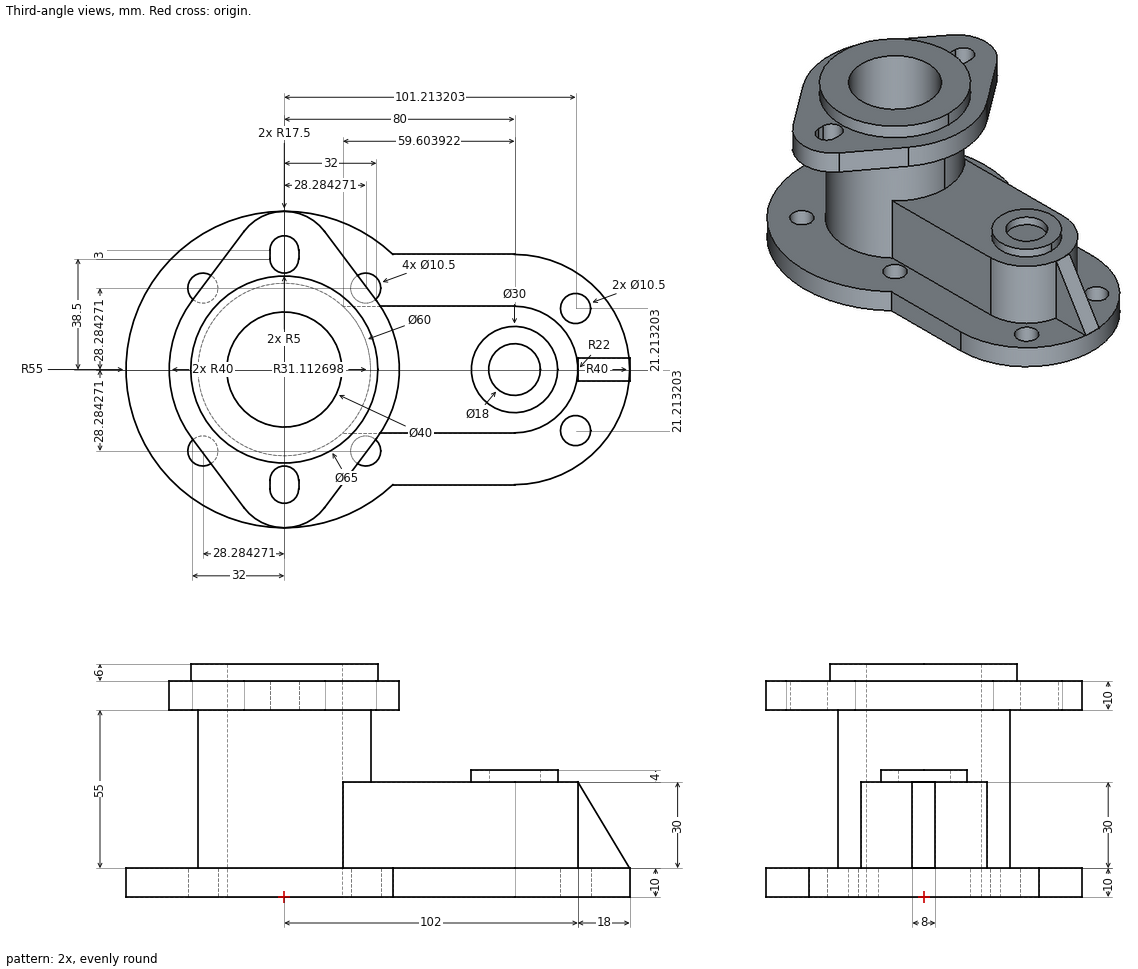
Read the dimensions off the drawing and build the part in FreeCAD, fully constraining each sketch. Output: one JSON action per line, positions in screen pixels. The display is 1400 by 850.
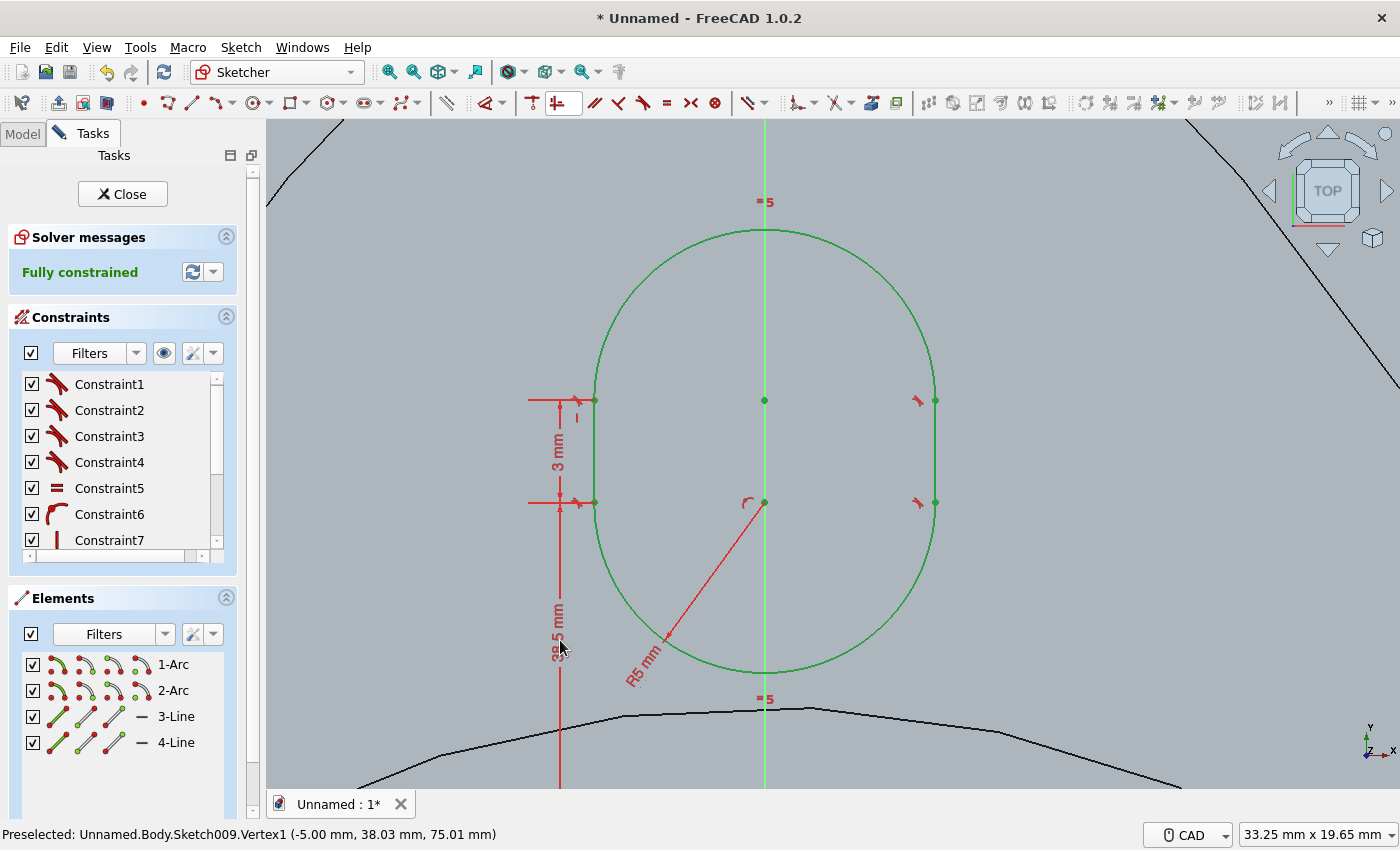
{"action": "left_click", "coordinate": [123, 194]}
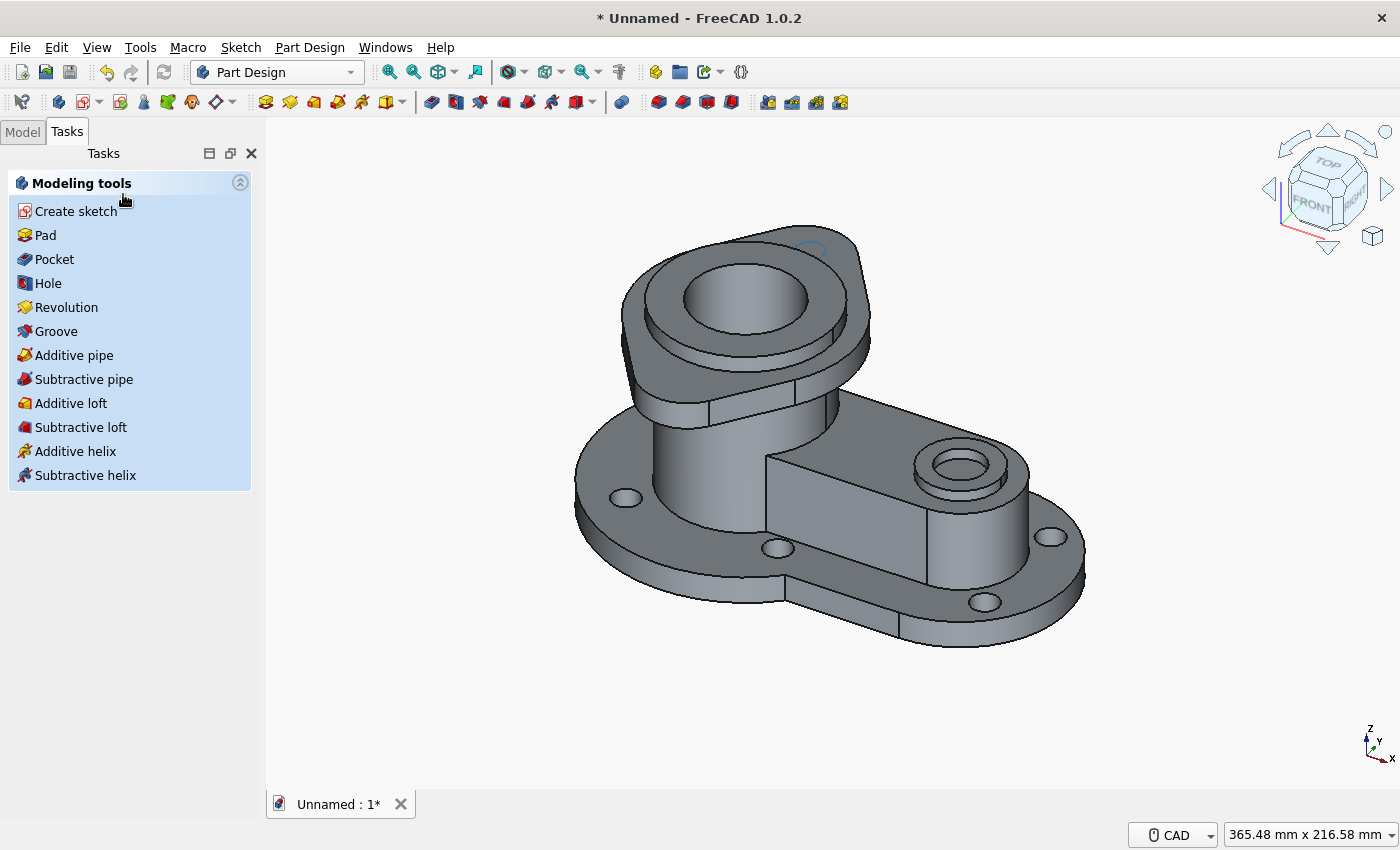
{"action": "left_click", "coordinate": [432, 102]}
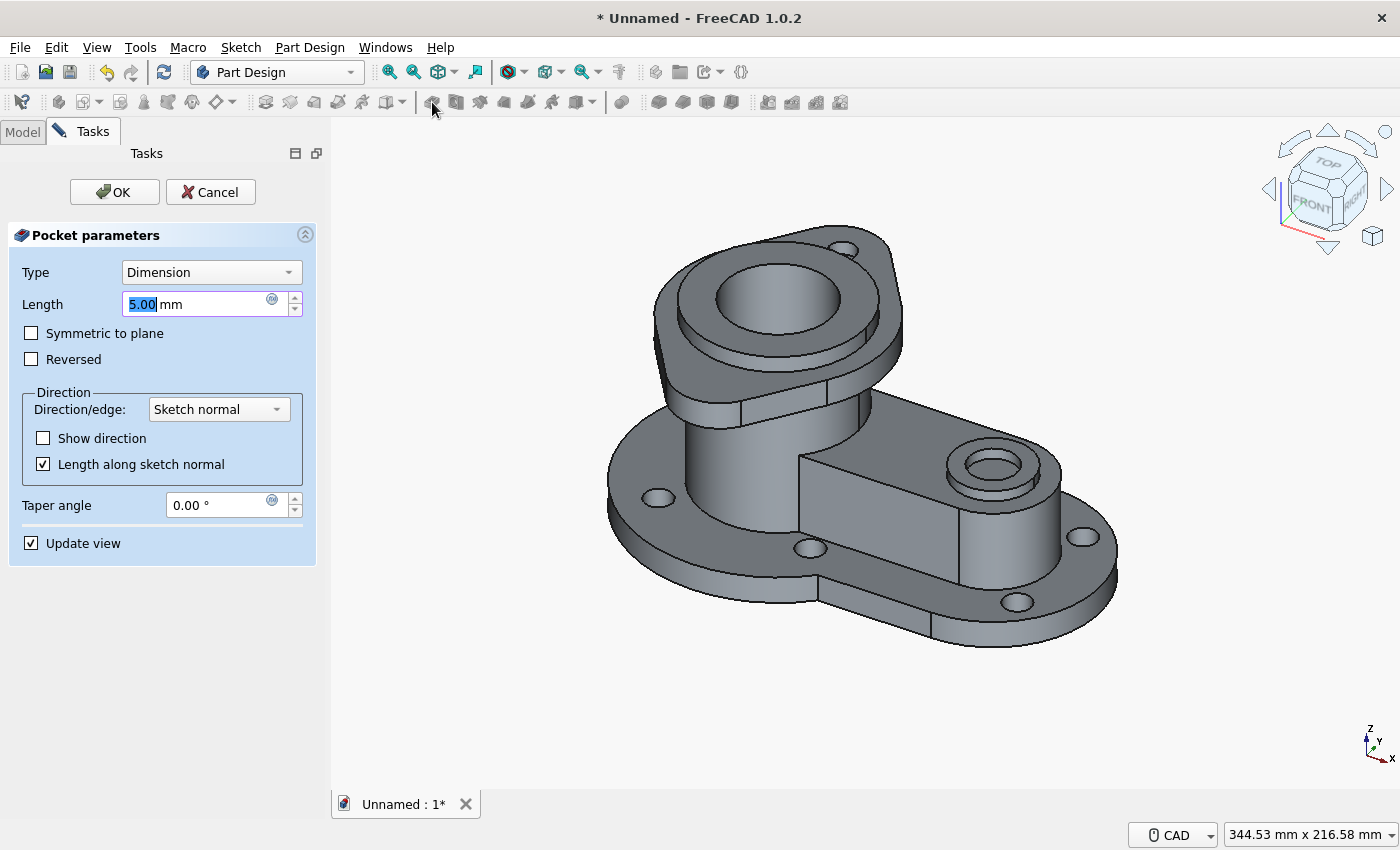
{"action": "type", "text": "10"}
{"action": "key", "text": "Tab"}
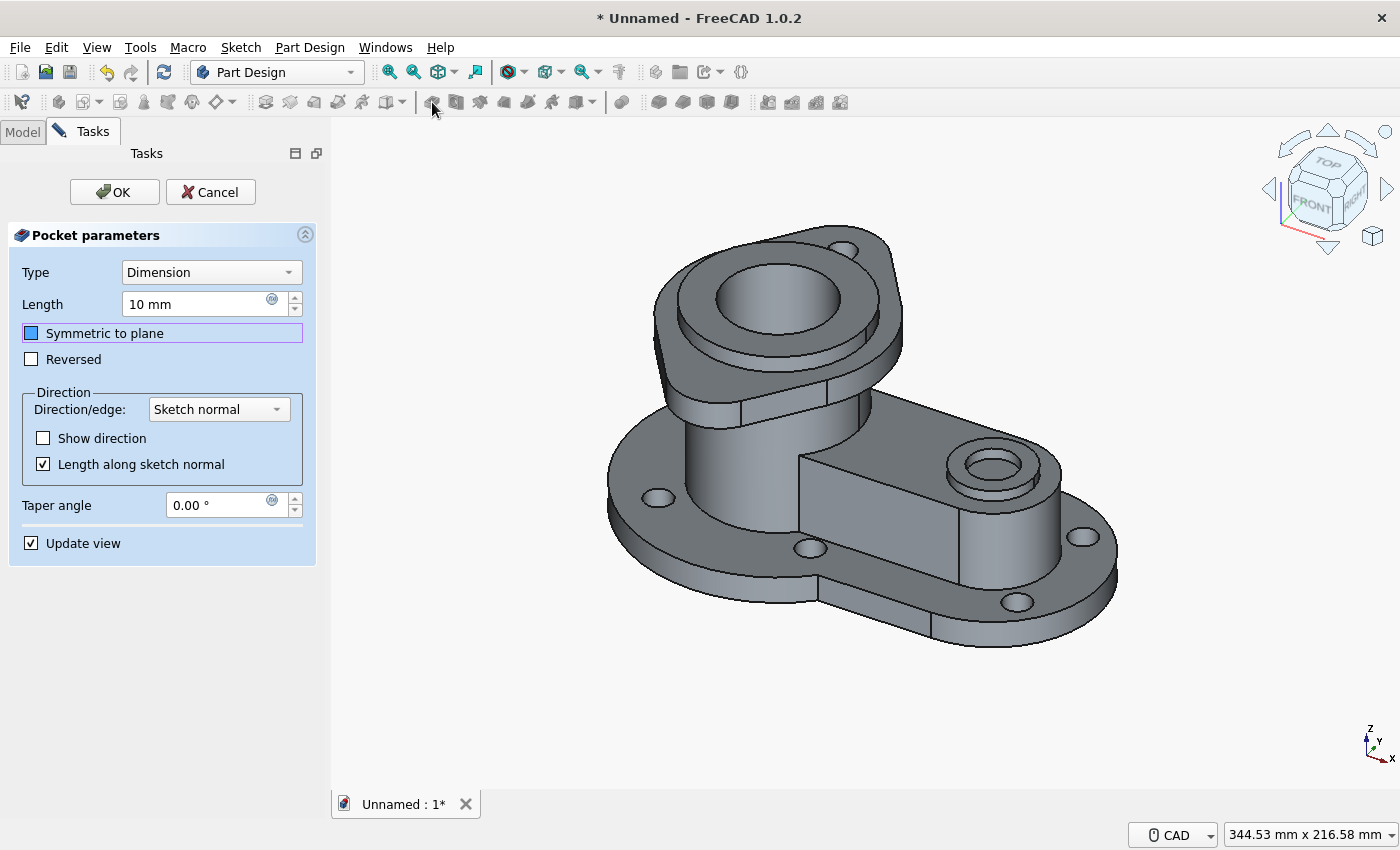
{"action": "left_click", "coordinate": [115, 192]}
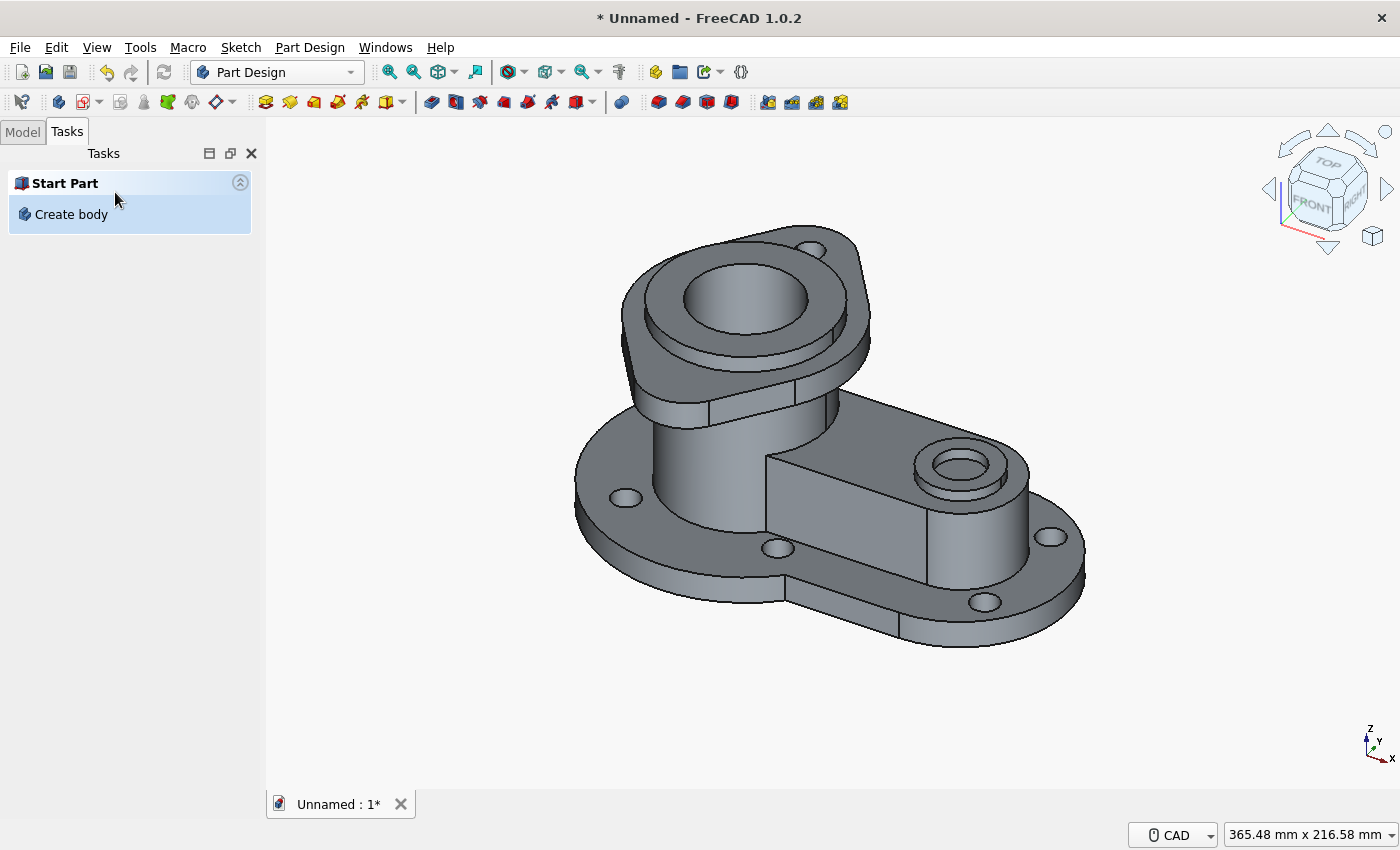
{"action": "left_click", "coordinate": [23, 131]}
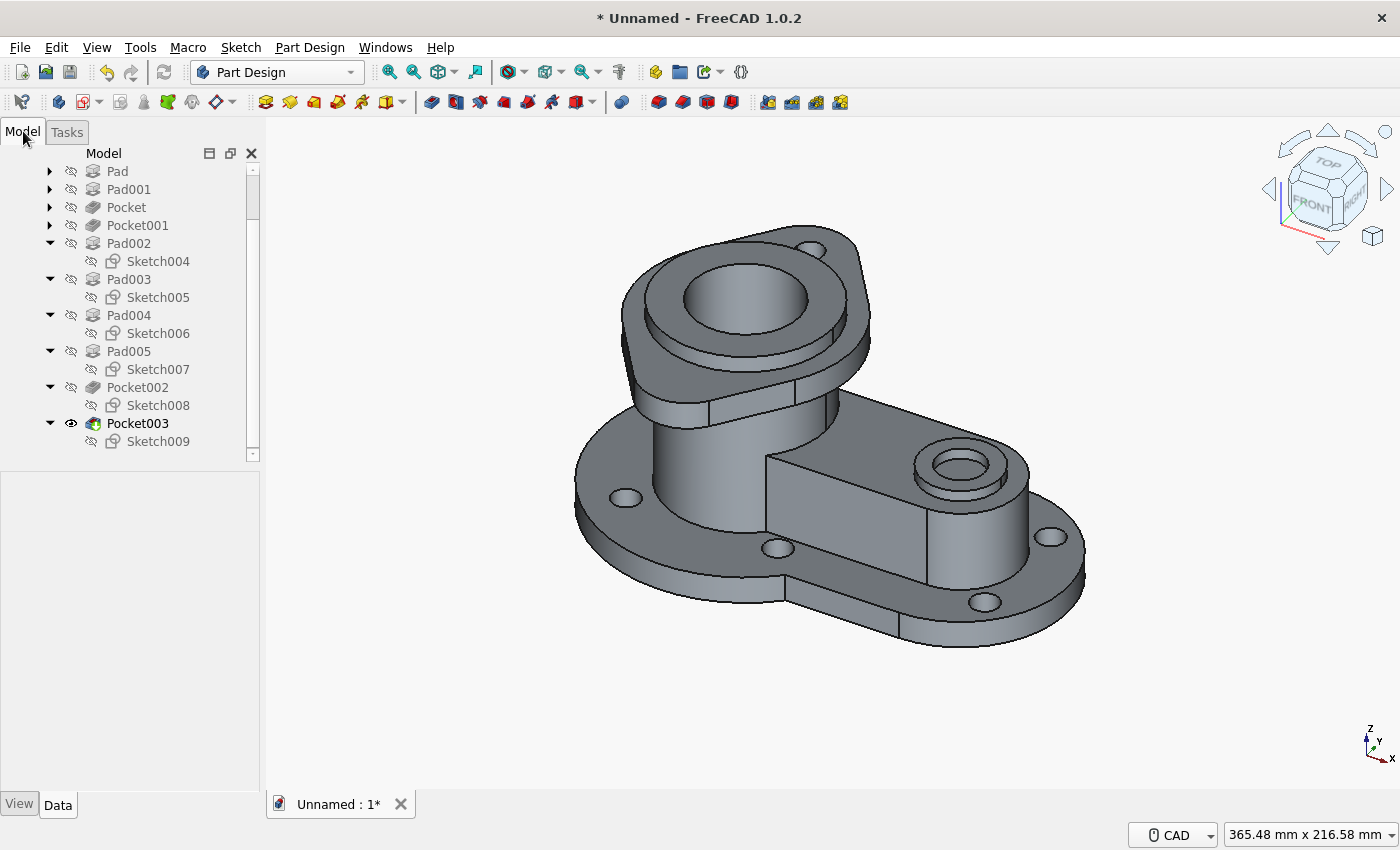
{"action": "left_click", "coordinate": [116, 423]}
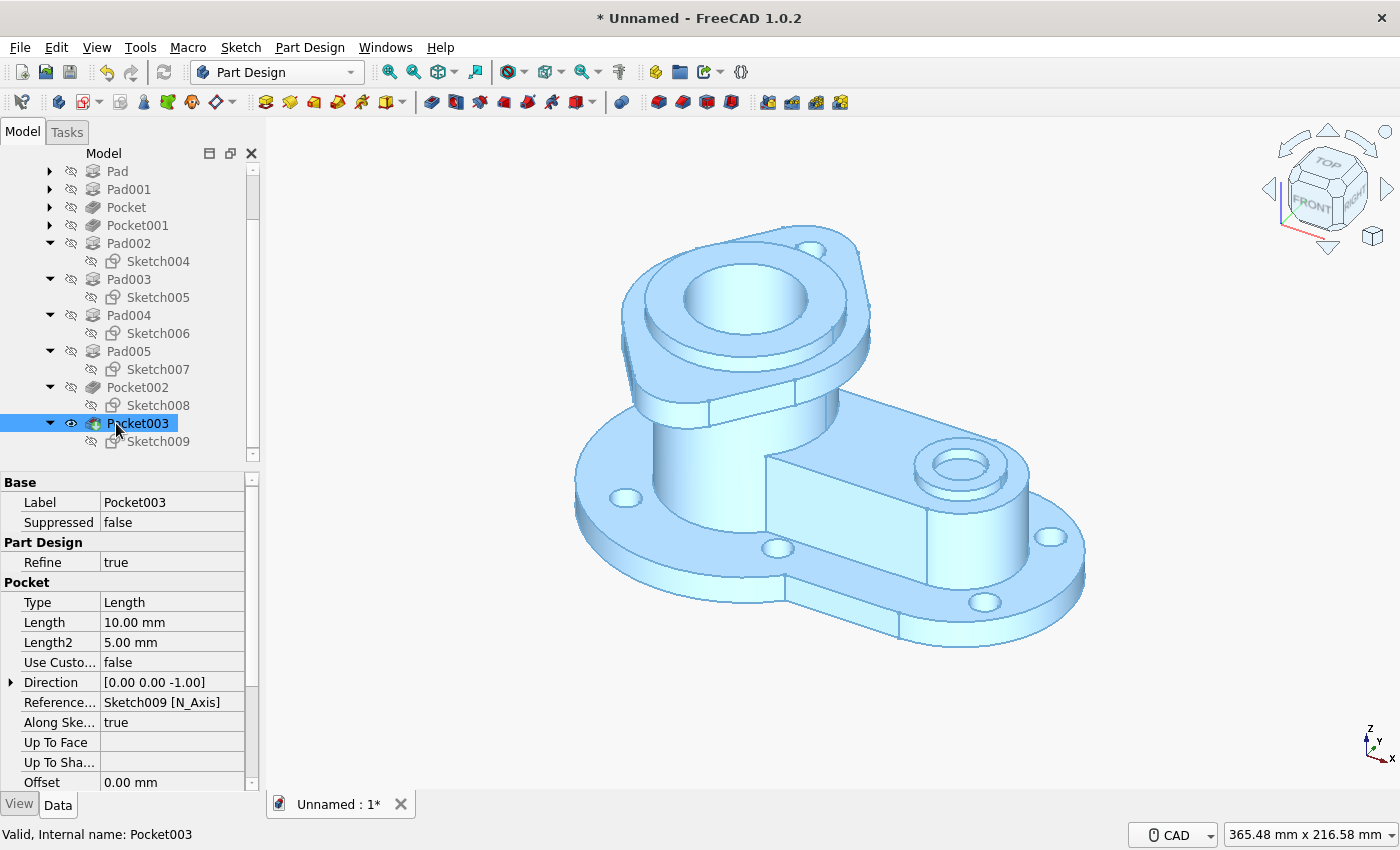
{"action": "left_click", "coordinate": [816, 102]}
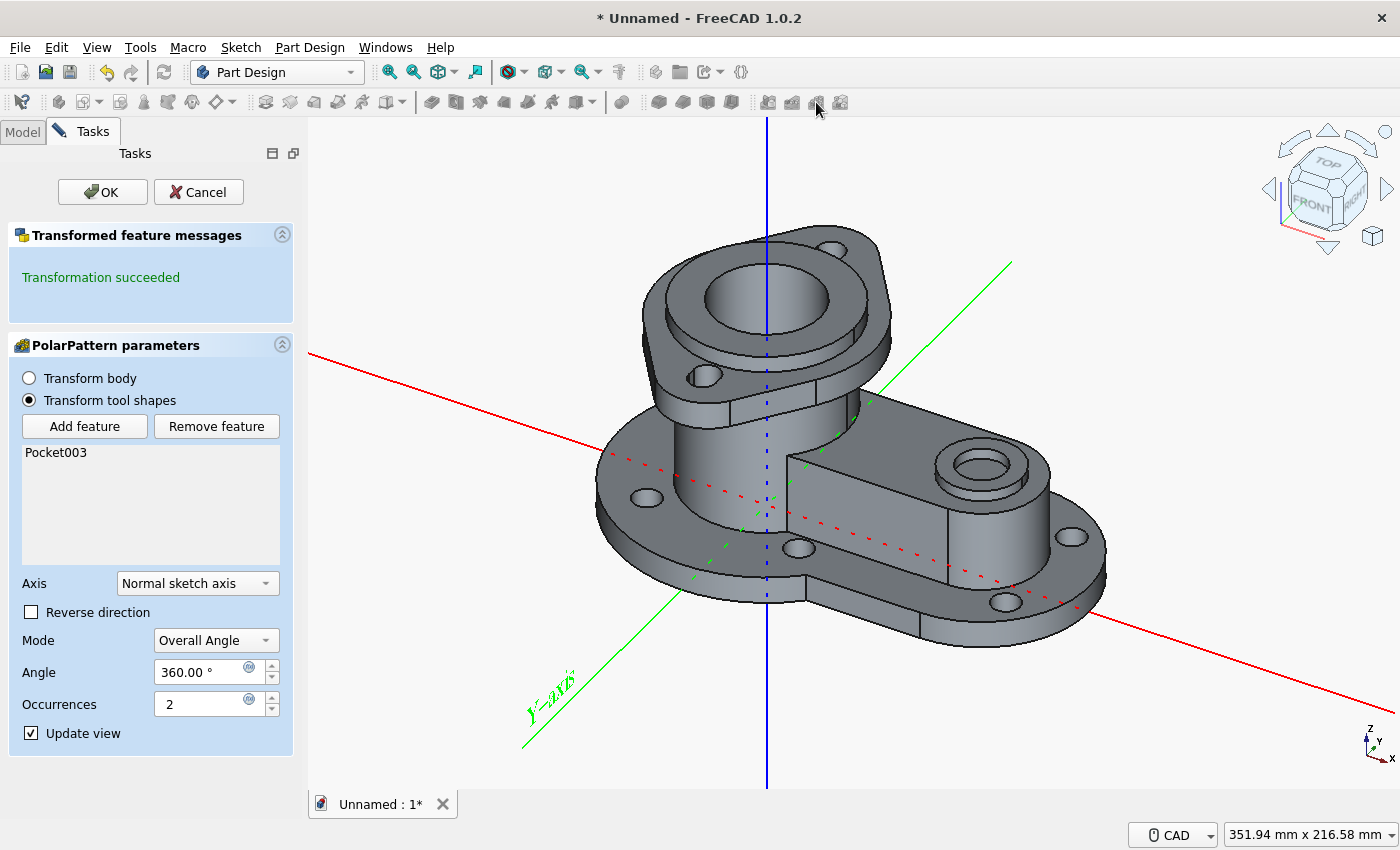
{"action": "left_click", "coordinate": [198, 584]}